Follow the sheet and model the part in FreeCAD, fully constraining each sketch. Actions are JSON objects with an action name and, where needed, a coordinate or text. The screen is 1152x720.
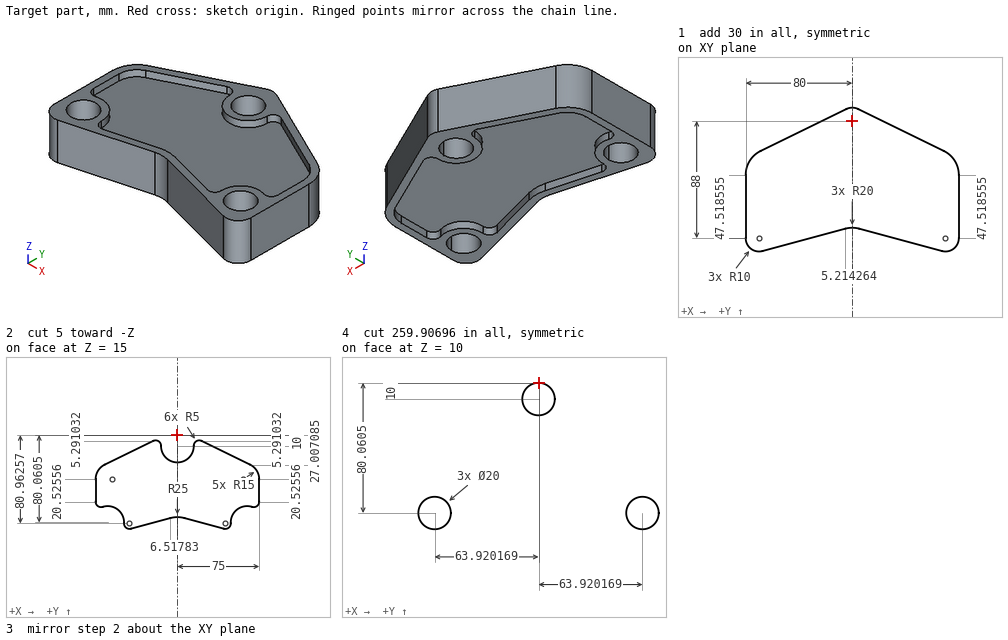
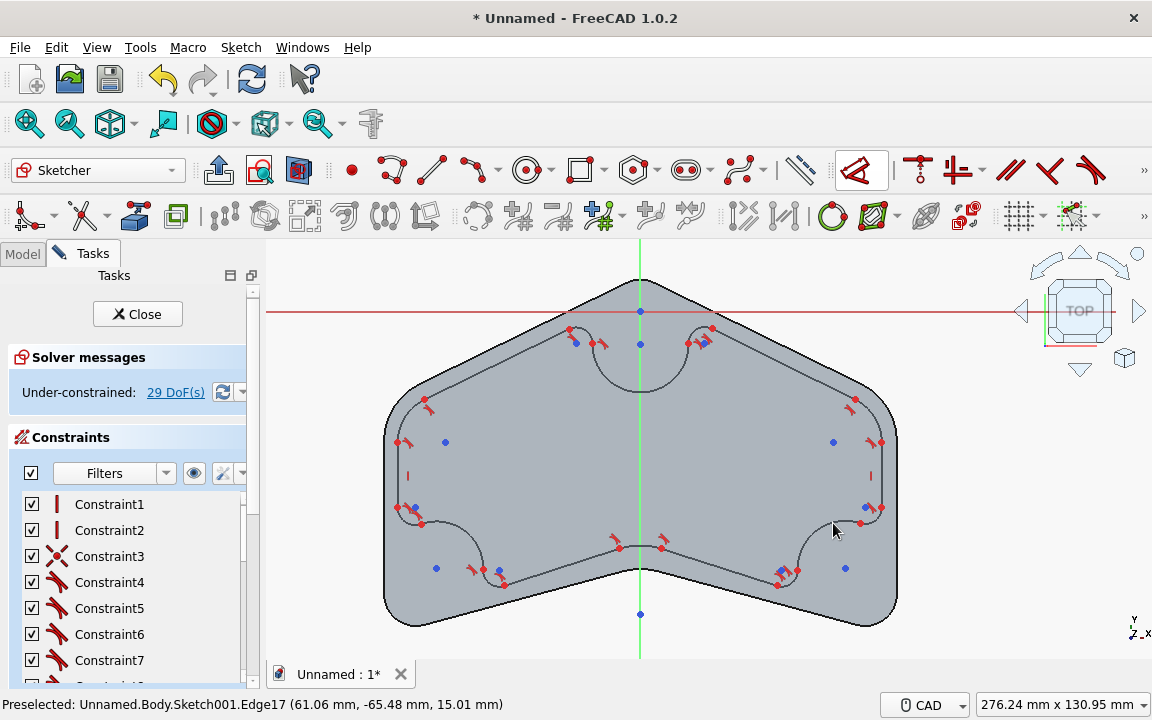
{"action": "left_click", "coordinate": [833, 523]}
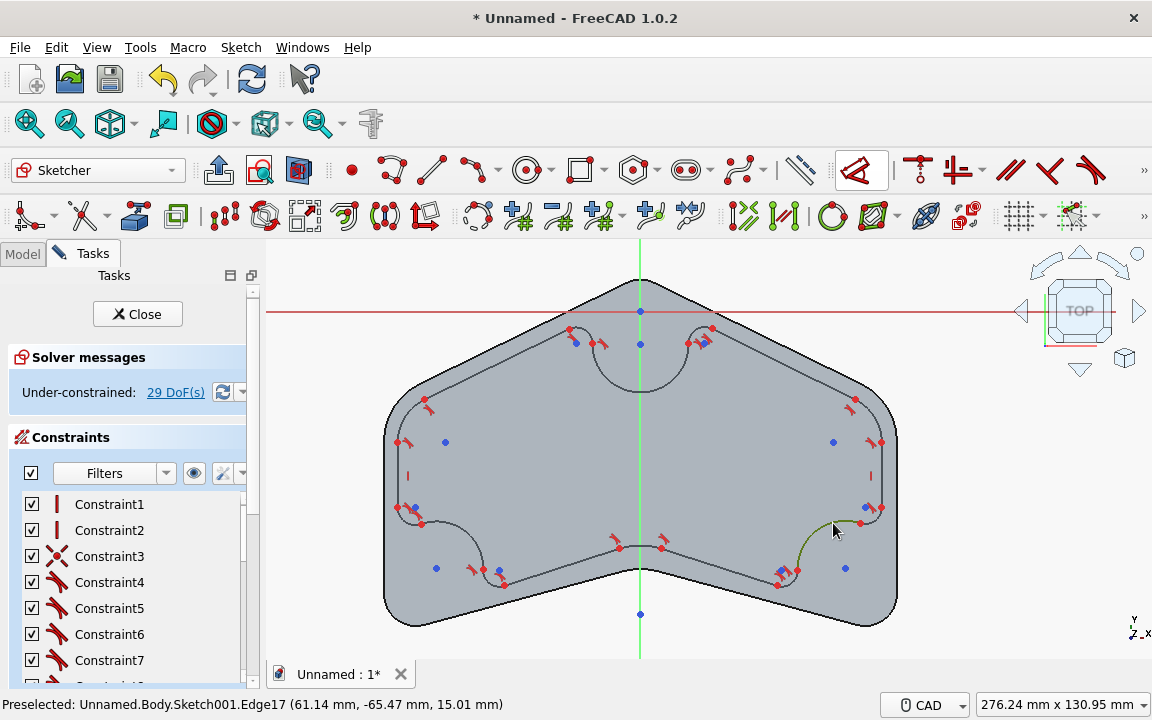
{"action": "scroll", "coordinate": [869, 524], "scroll_direction": "up", "scroll_amount": 3}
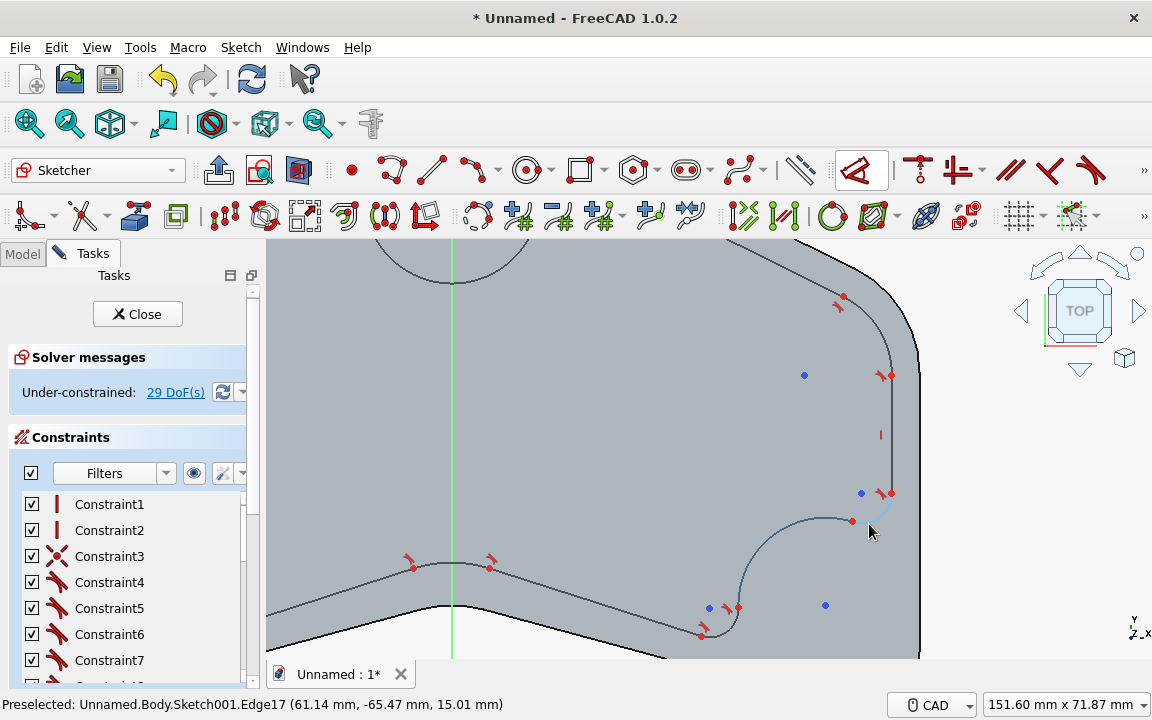
{"action": "left_click", "coordinate": [869, 523]}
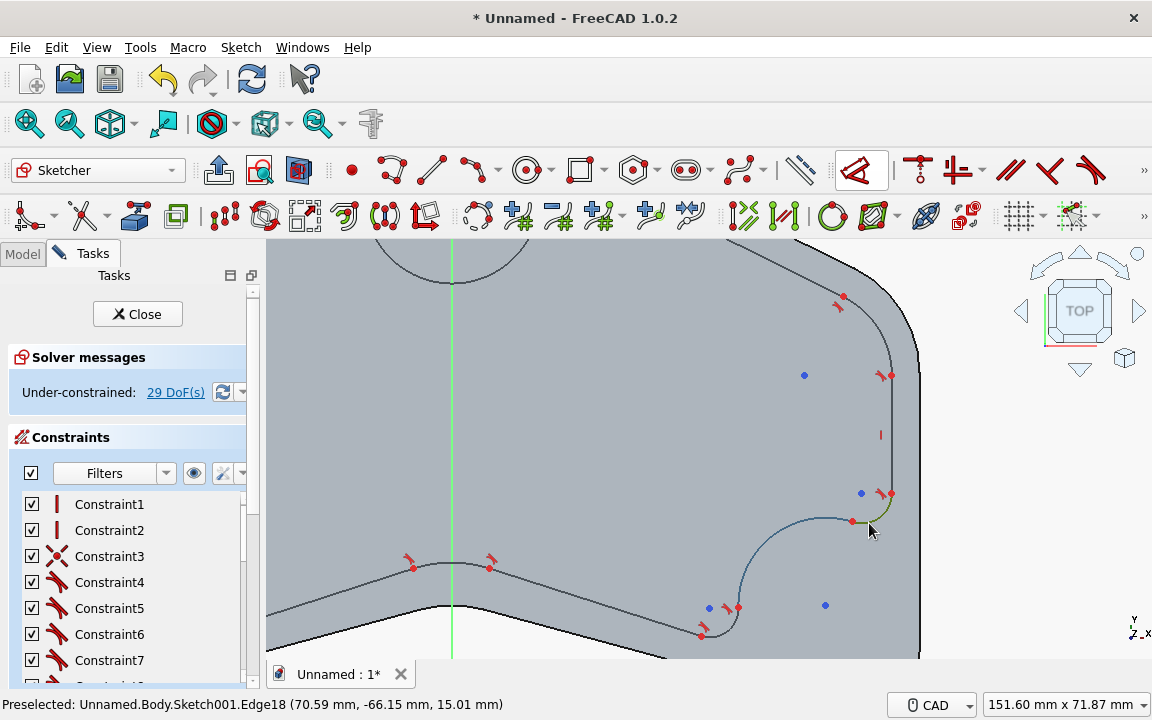
{"action": "key", "text": "t"}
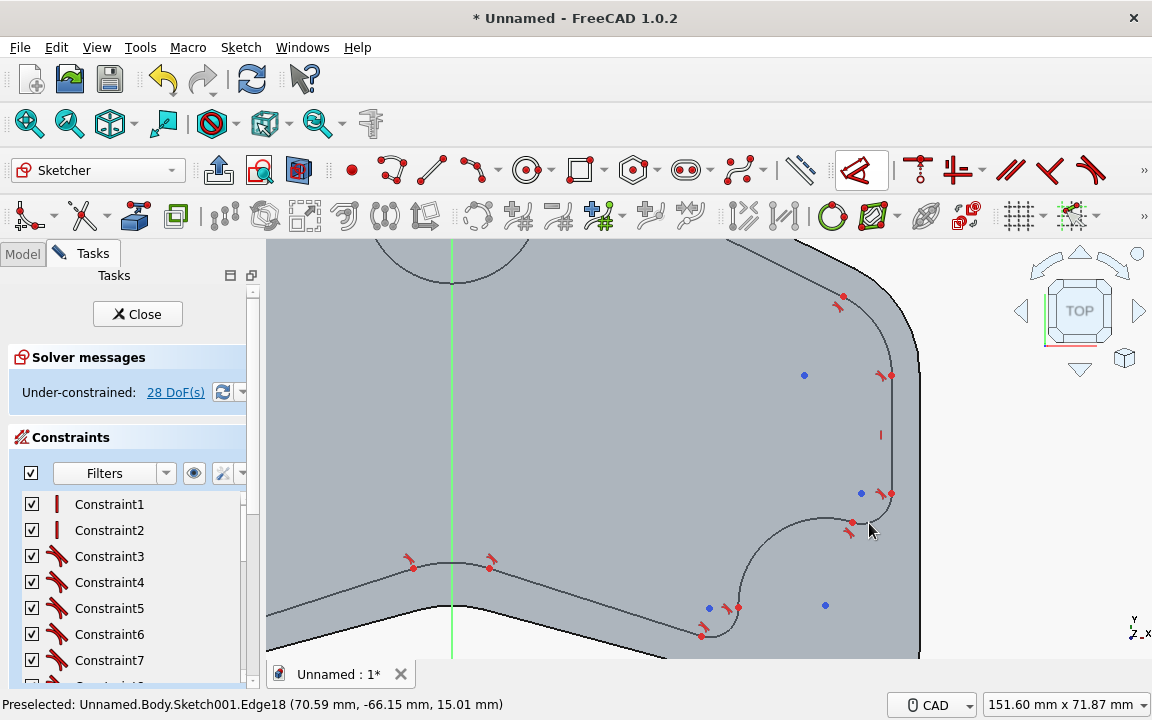
{"action": "left_click", "coordinate": [887, 347]}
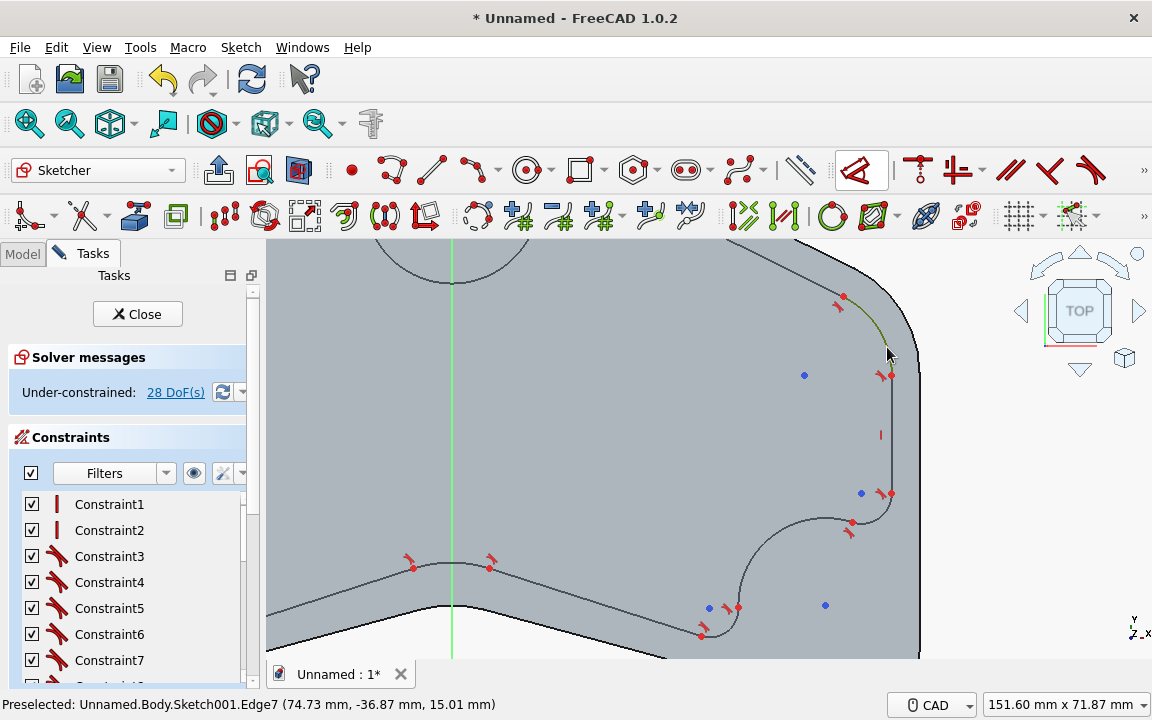
{"action": "left_click", "coordinate": [452, 284]}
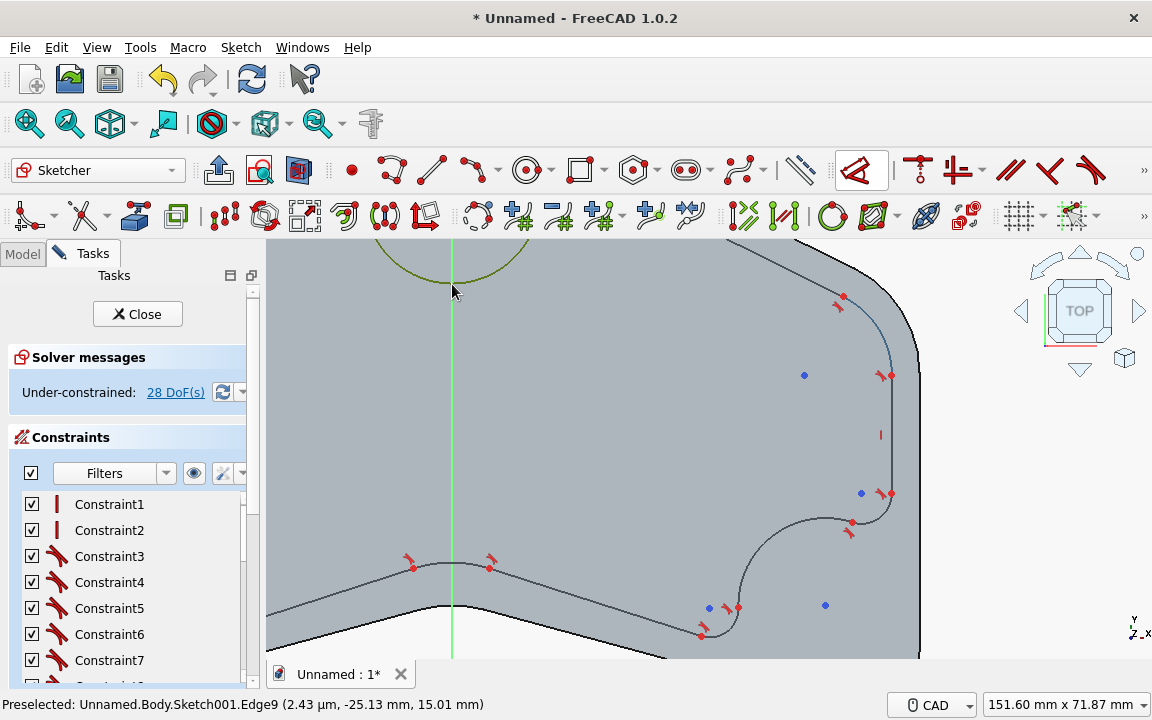
{"action": "scroll", "coordinate": [870, 524], "scroll_direction": "down", "scroll_amount": 3}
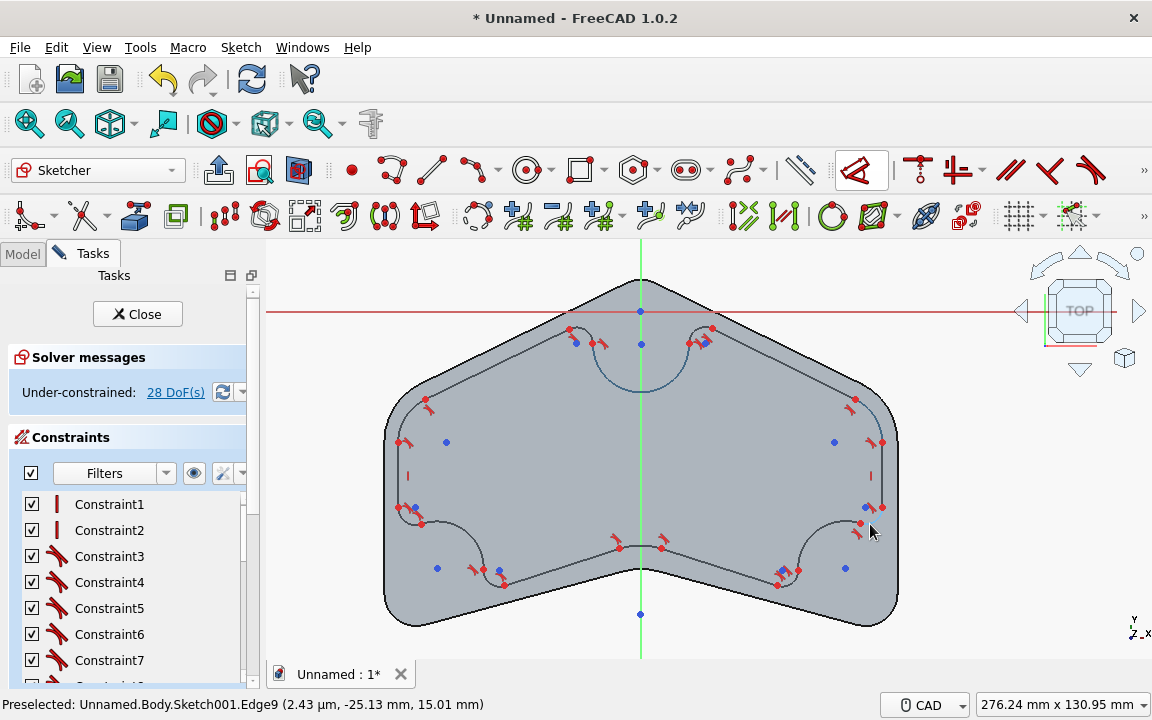
{"action": "left_click", "coordinate": [412, 409]}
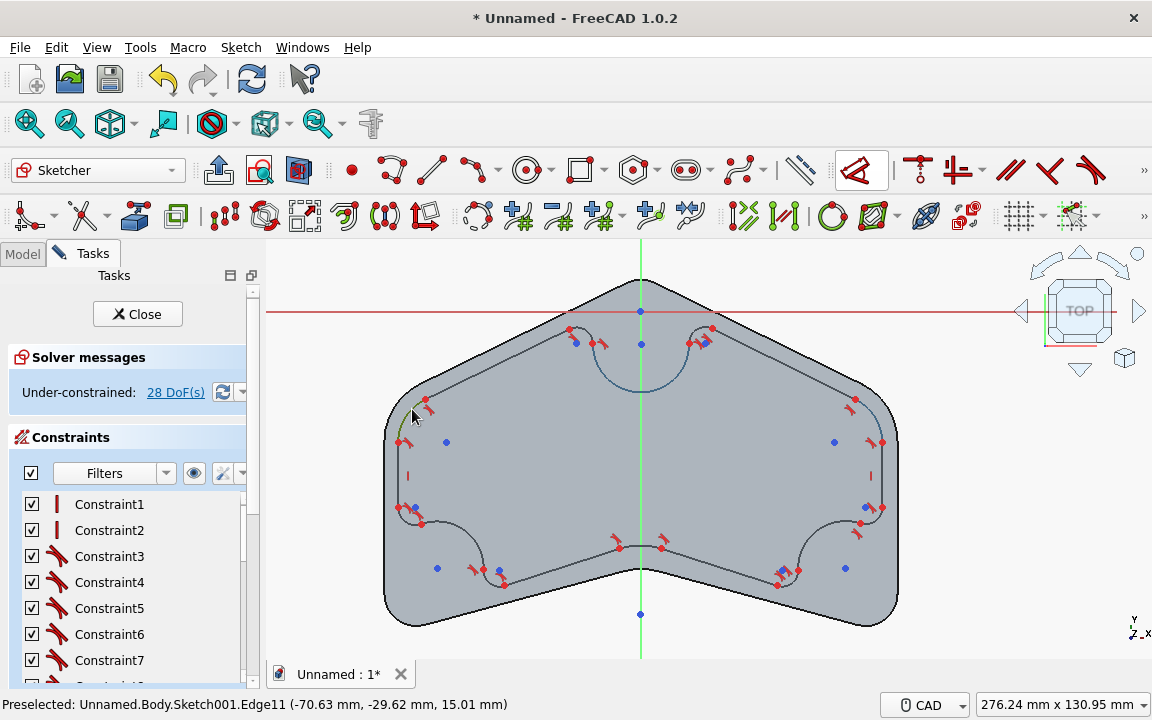
{"action": "left_click", "coordinate": [477, 544]}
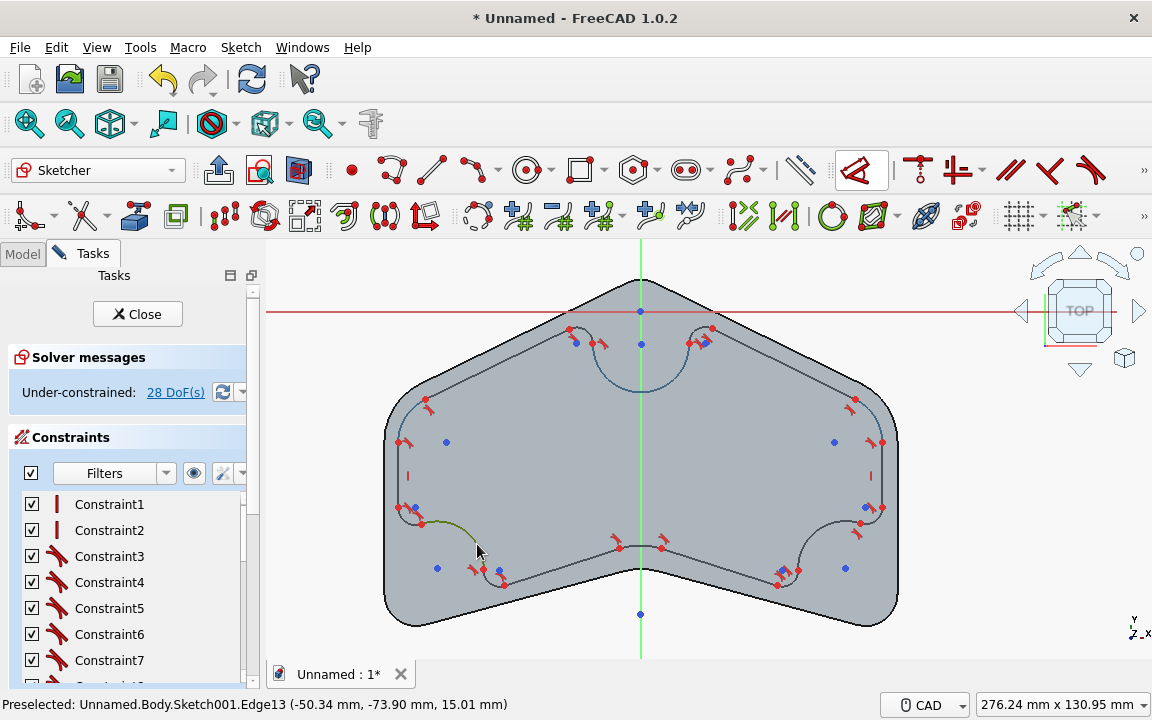
{"action": "left_click", "coordinate": [834, 523]}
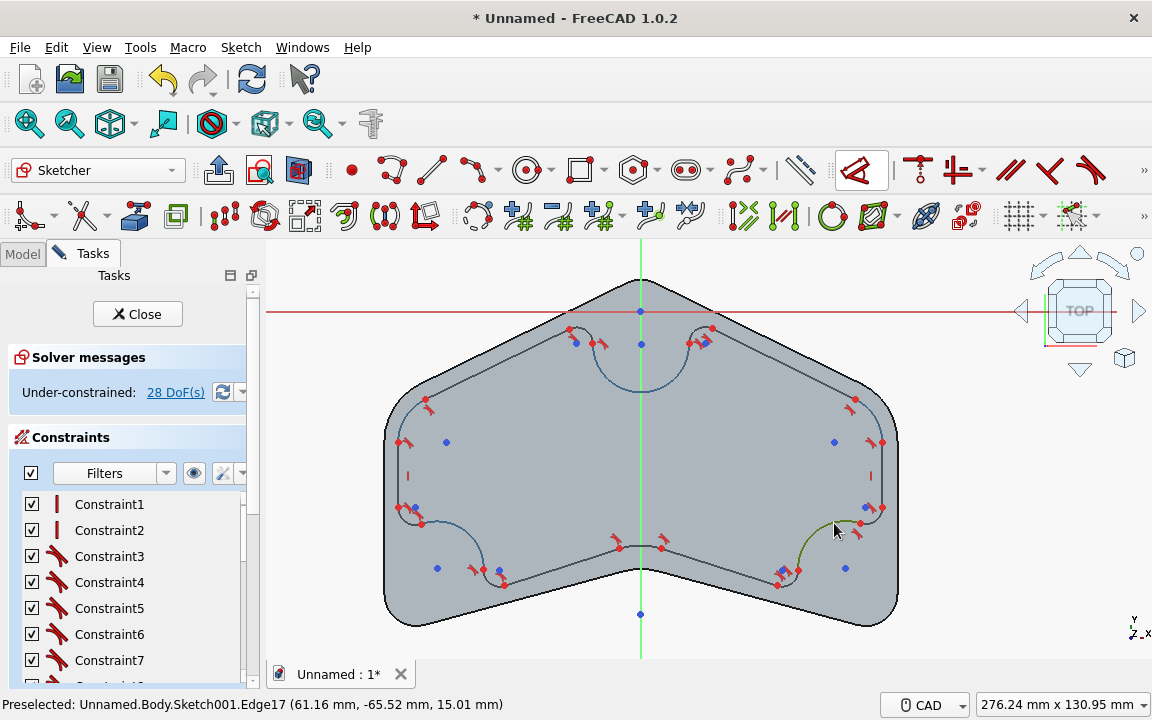
{"action": "key", "text": "e"}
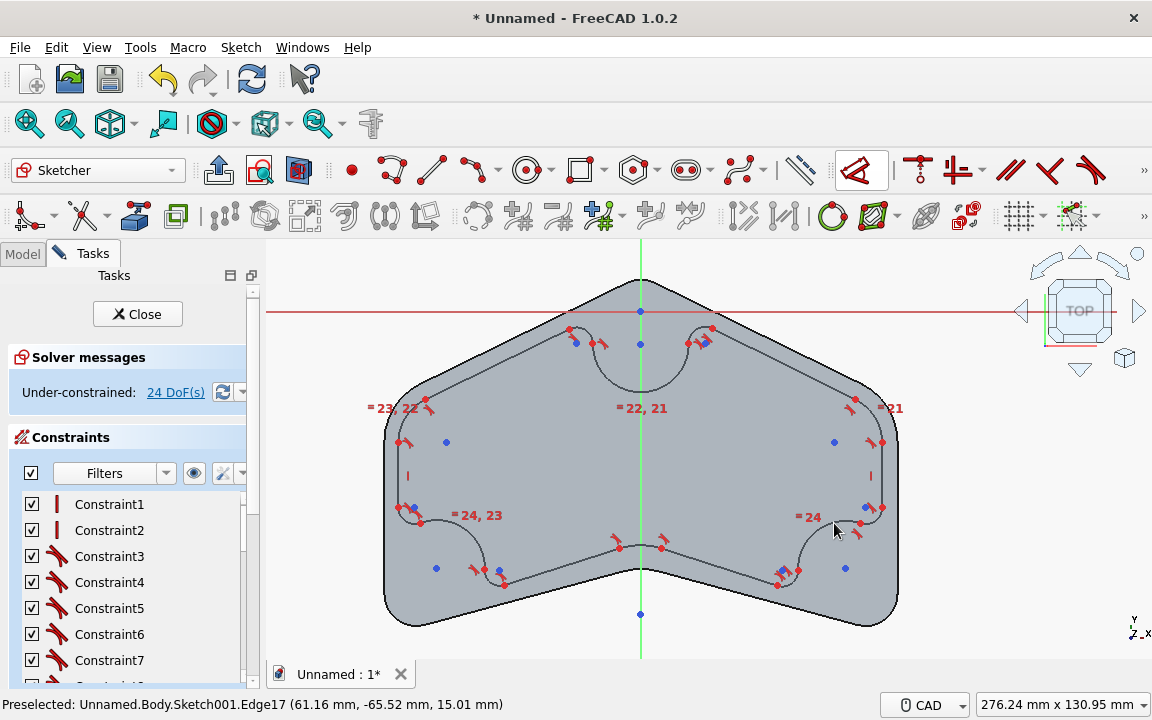
{"action": "scroll", "coordinate": [703, 327], "scroll_direction": "up", "scroll_amount": 2}